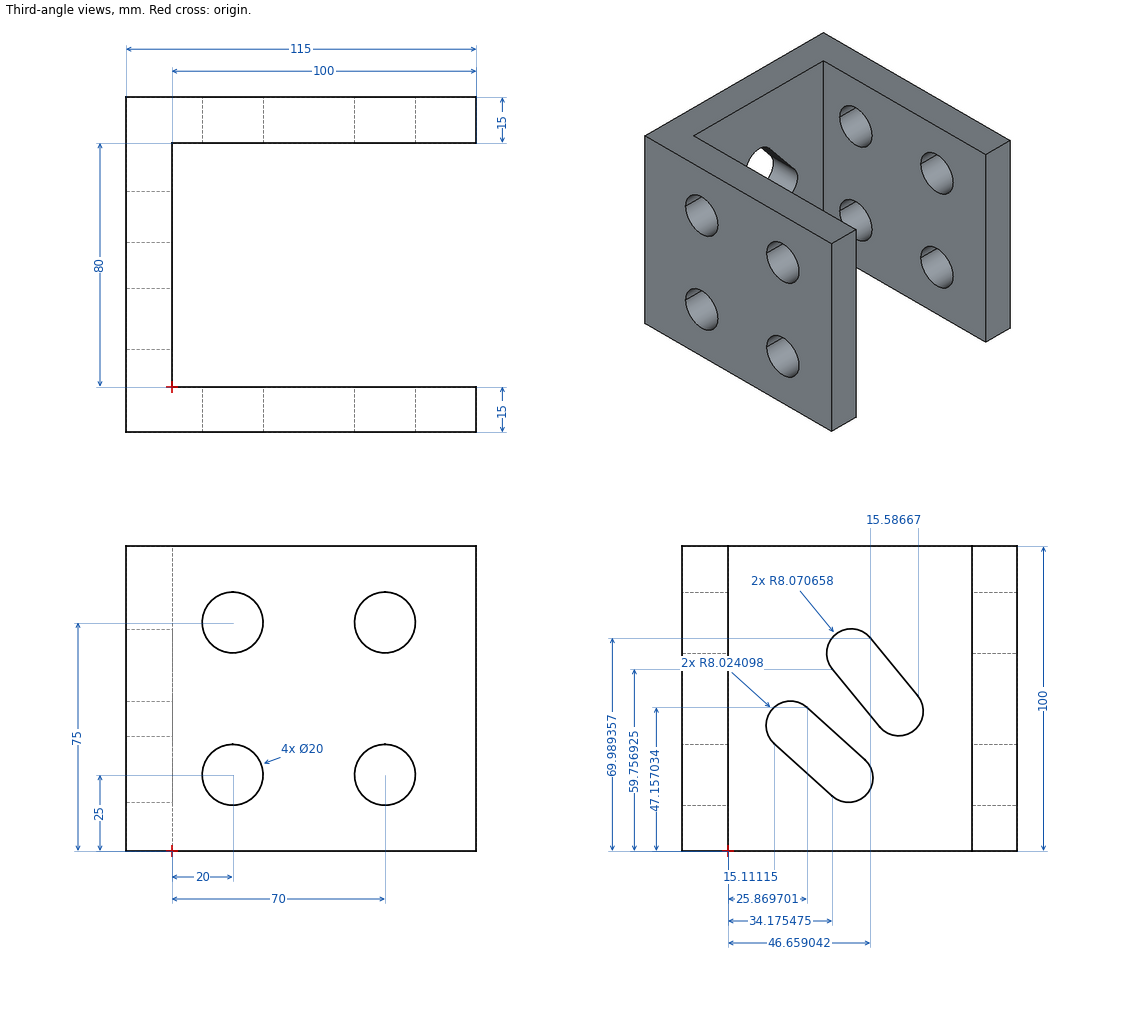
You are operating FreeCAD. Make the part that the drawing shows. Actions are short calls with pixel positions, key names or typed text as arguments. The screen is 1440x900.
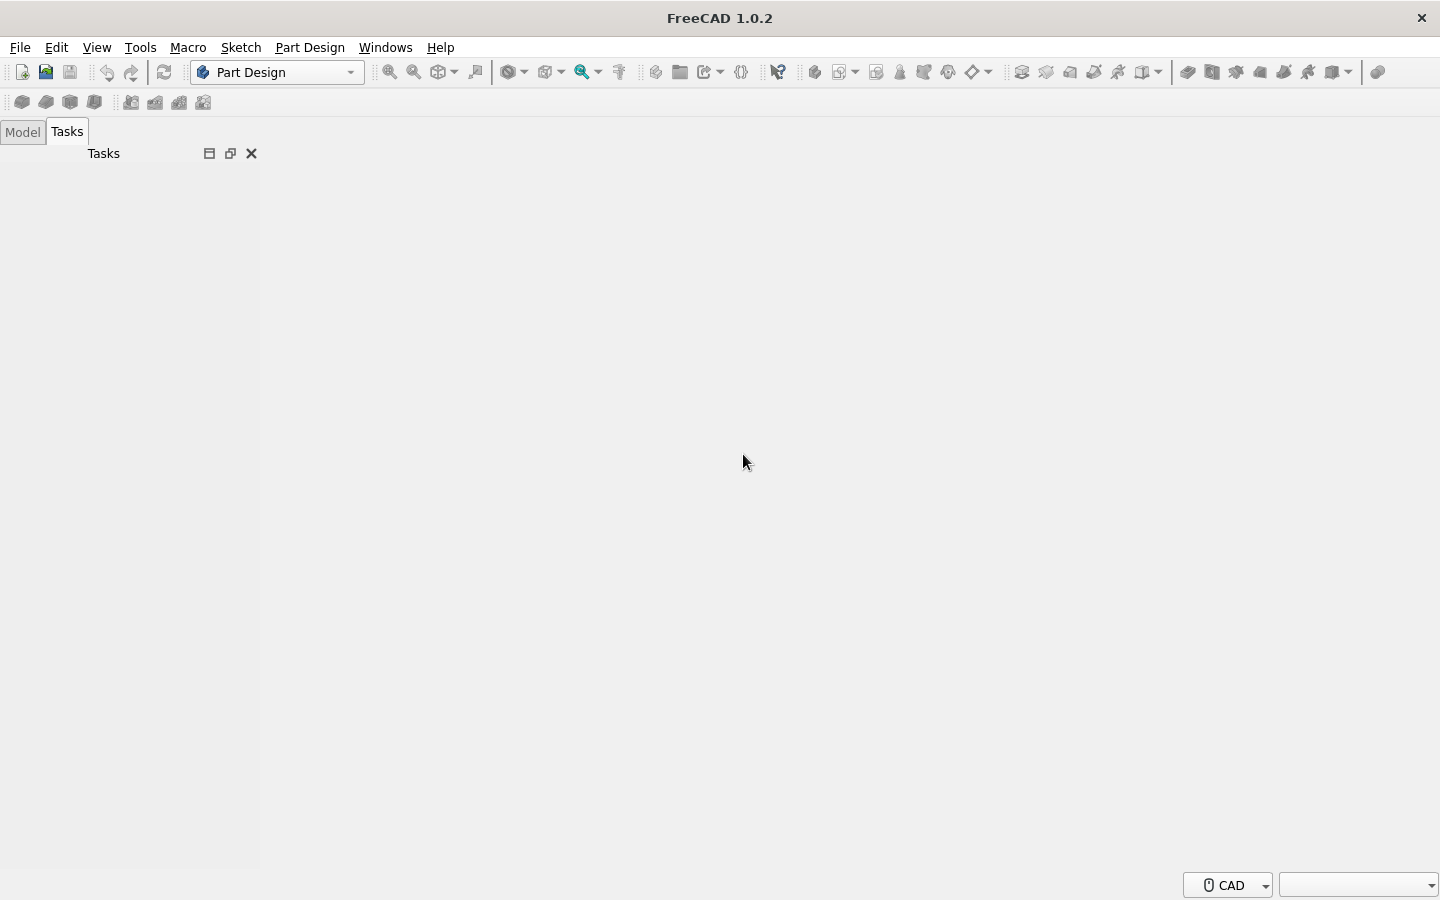
key(ctrl+n)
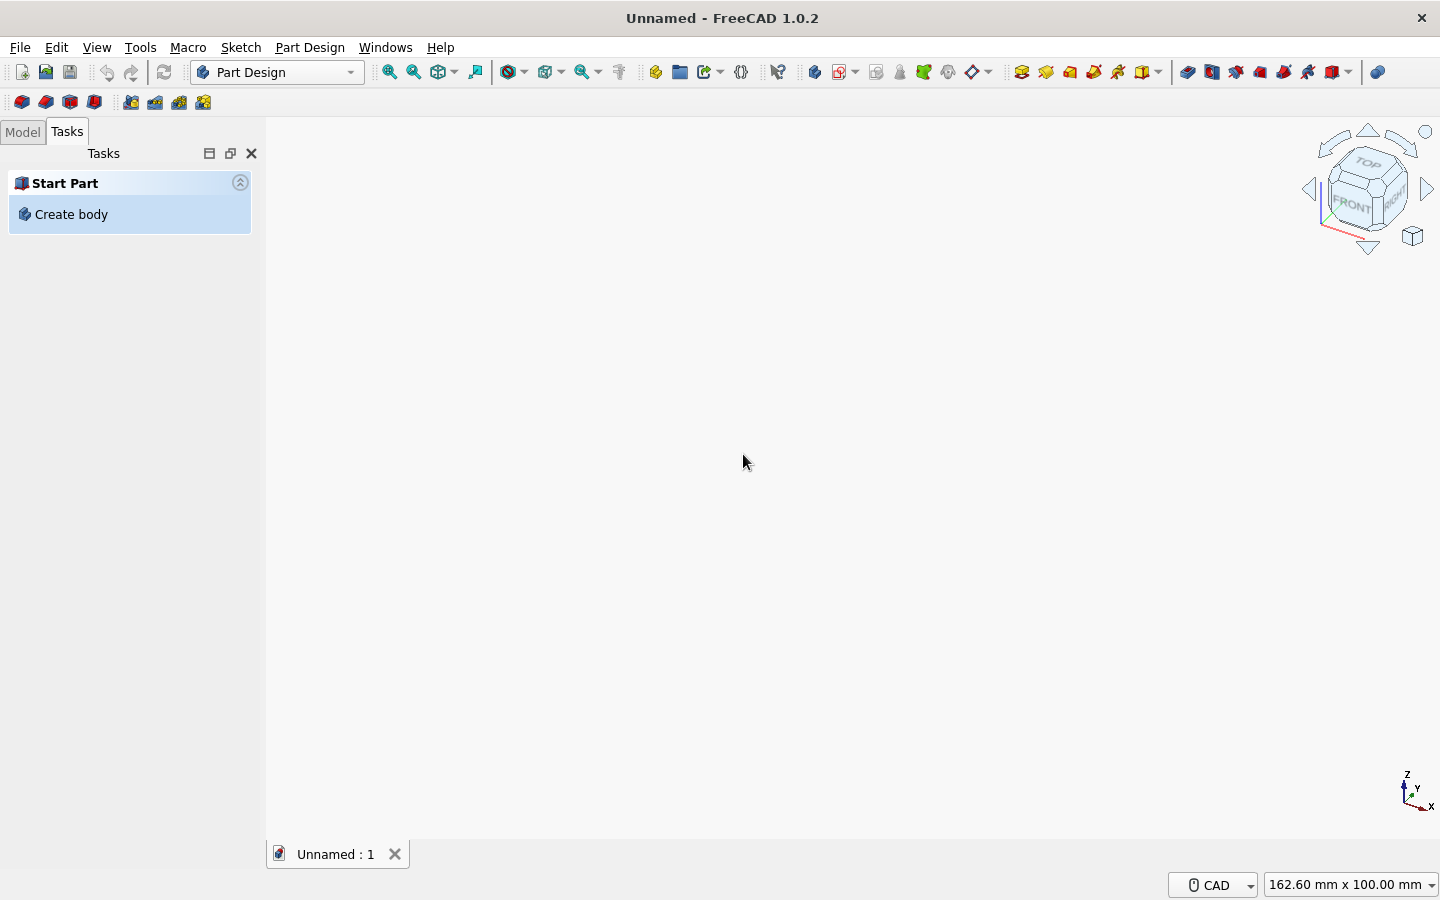
click(840, 72)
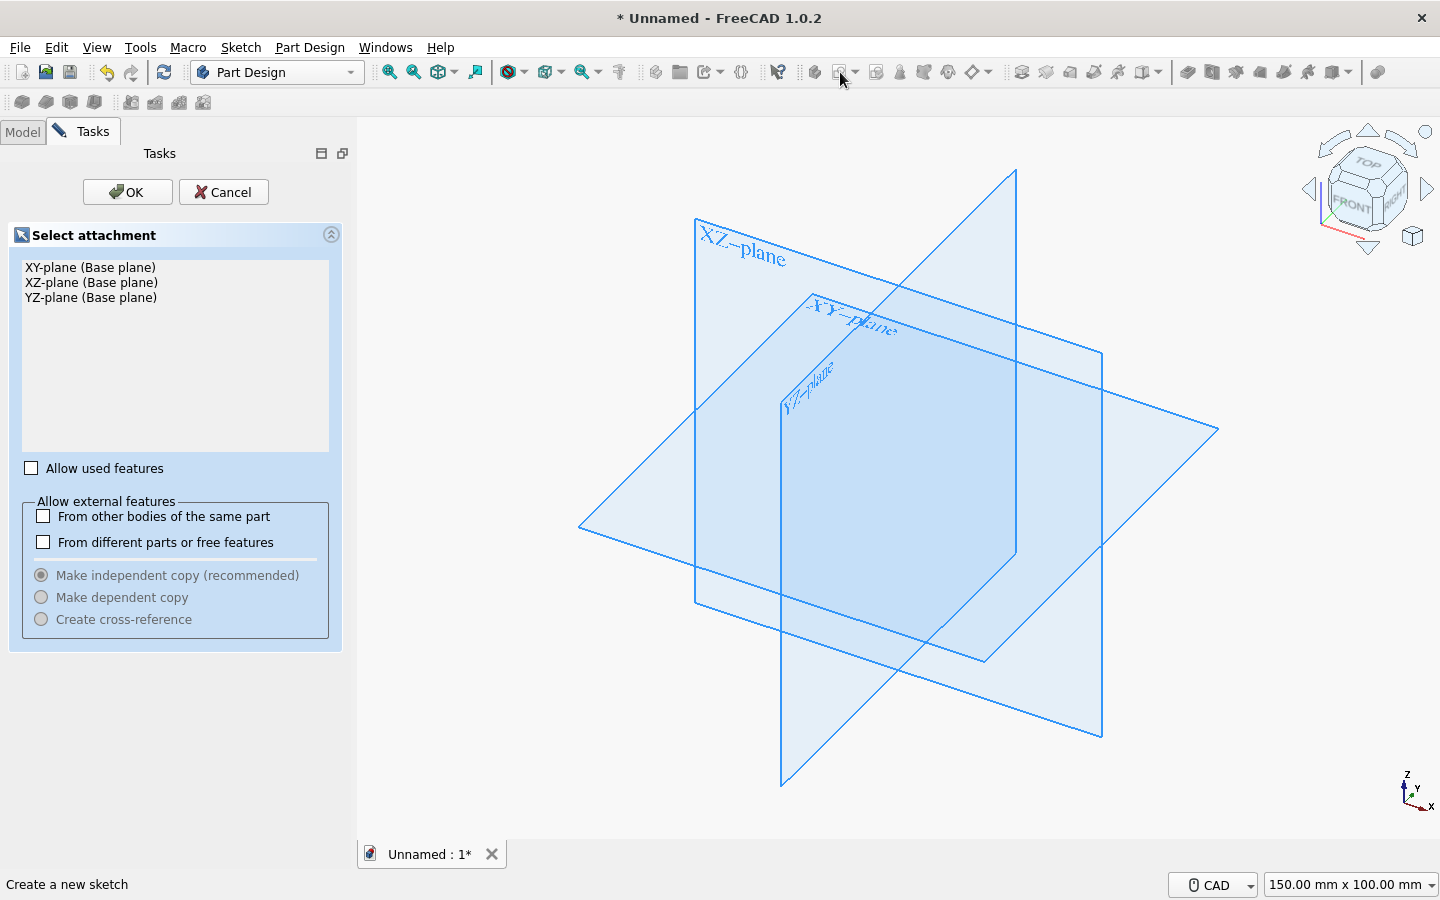
click(82, 268)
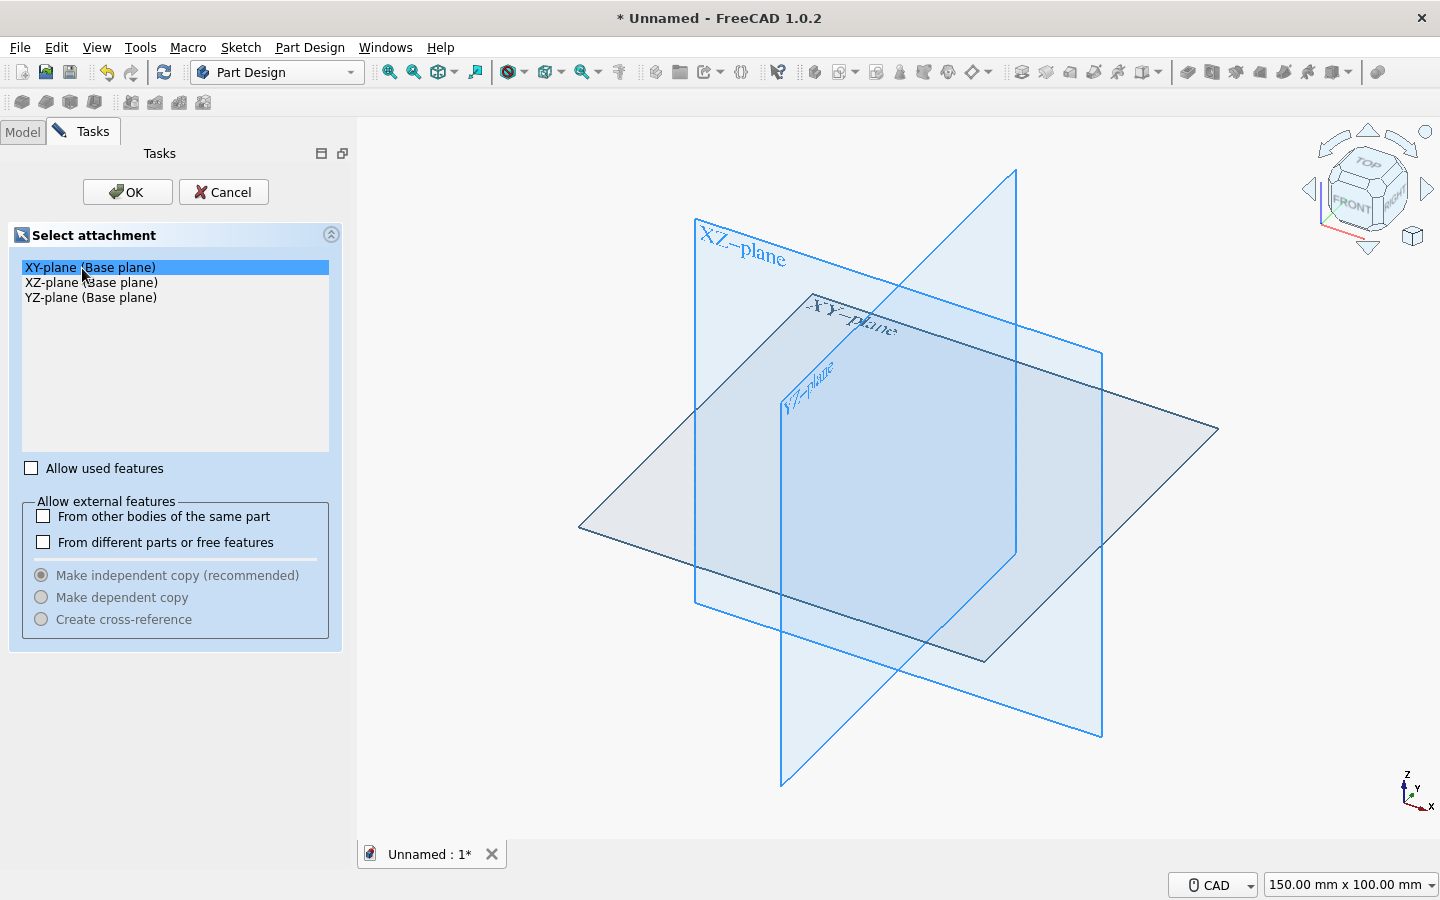
click(128, 192)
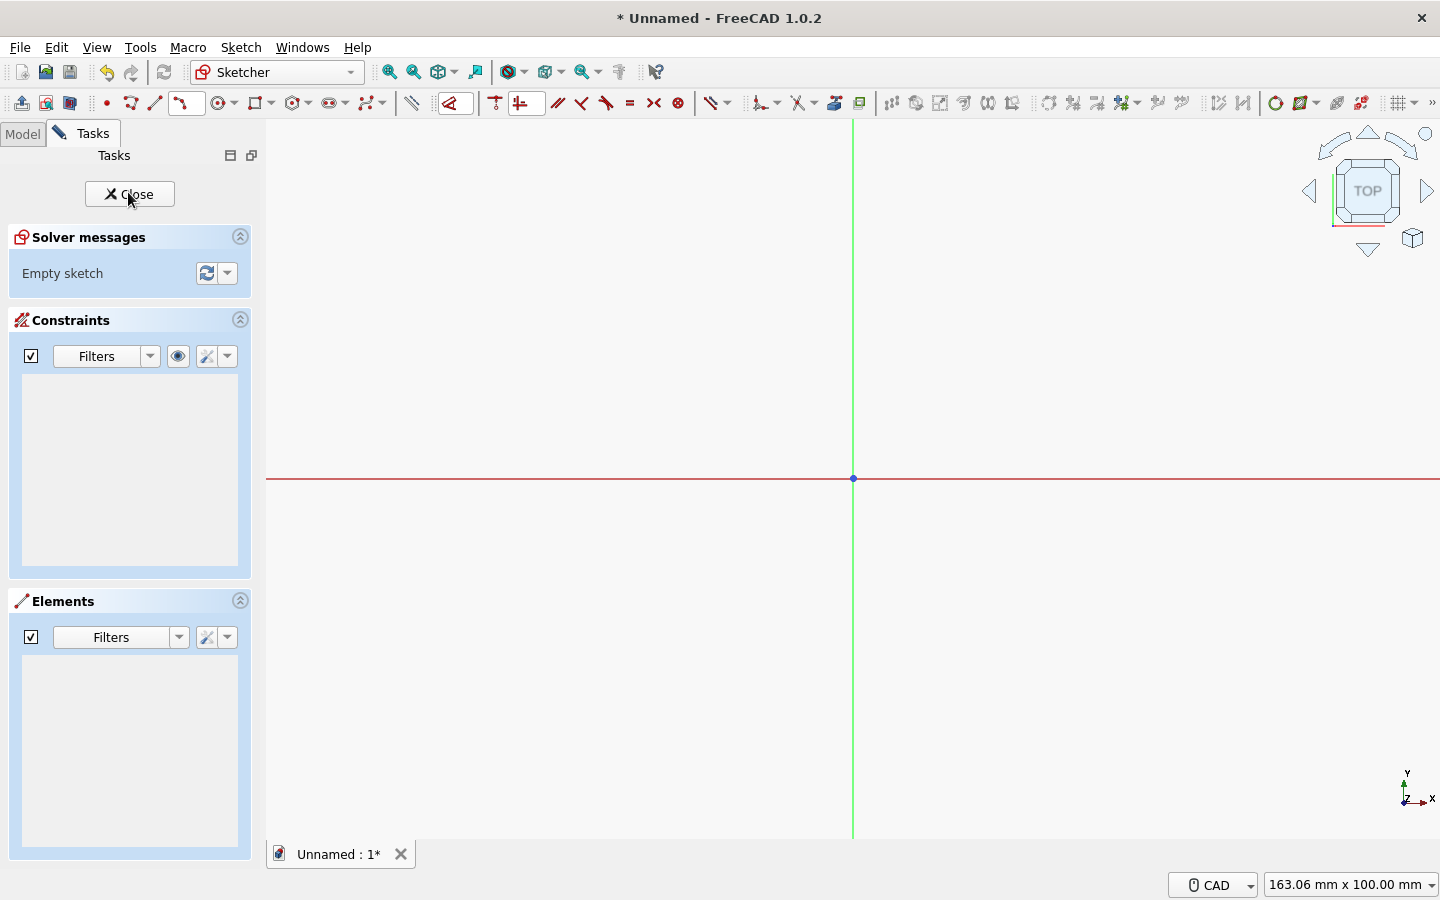
scroll(329, 811, down, 3)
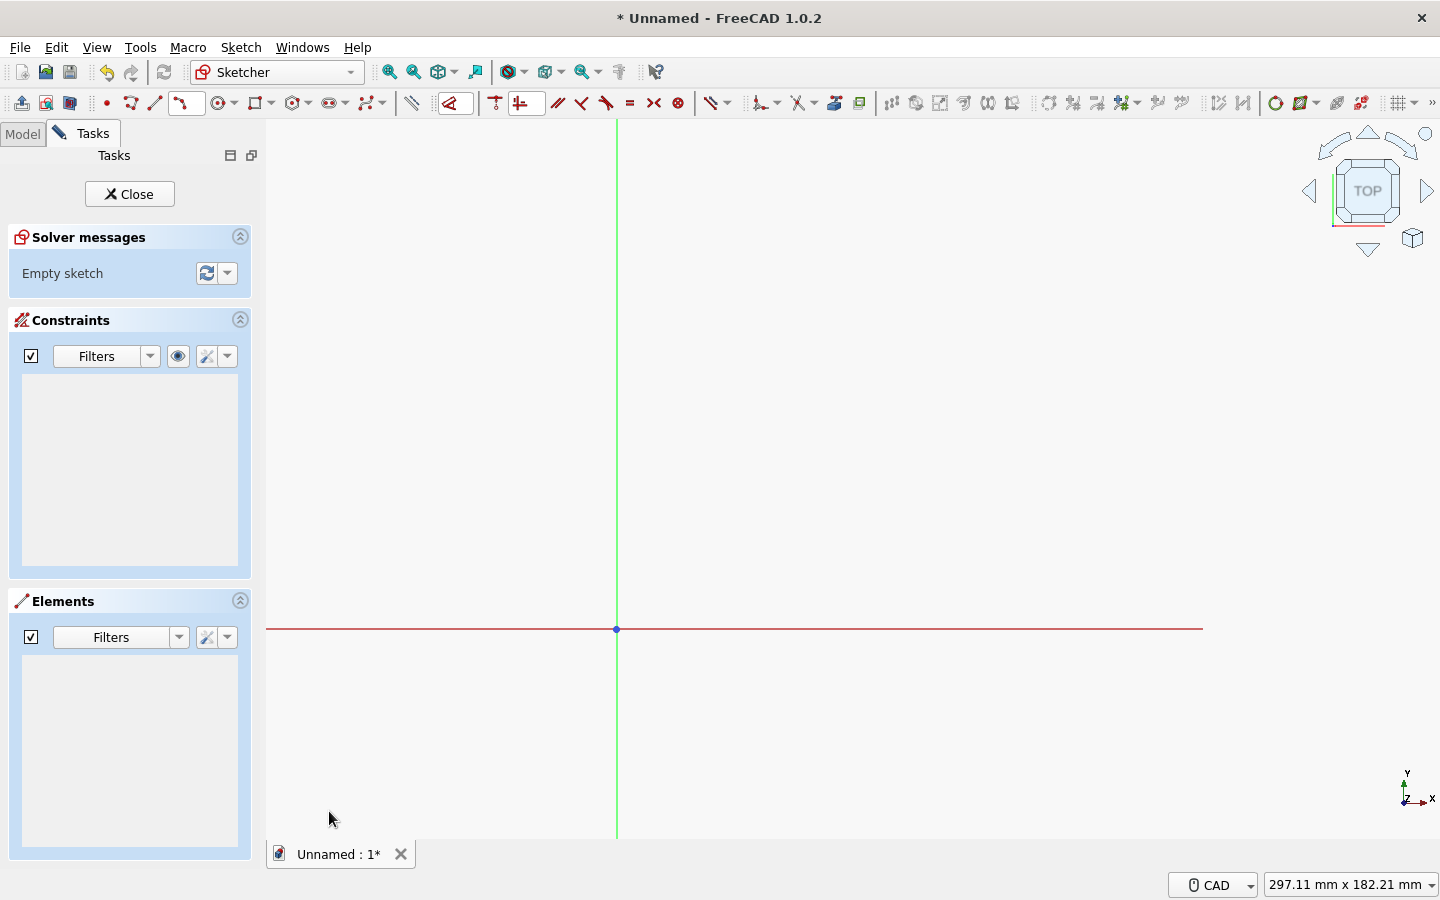
key(g)
key(m)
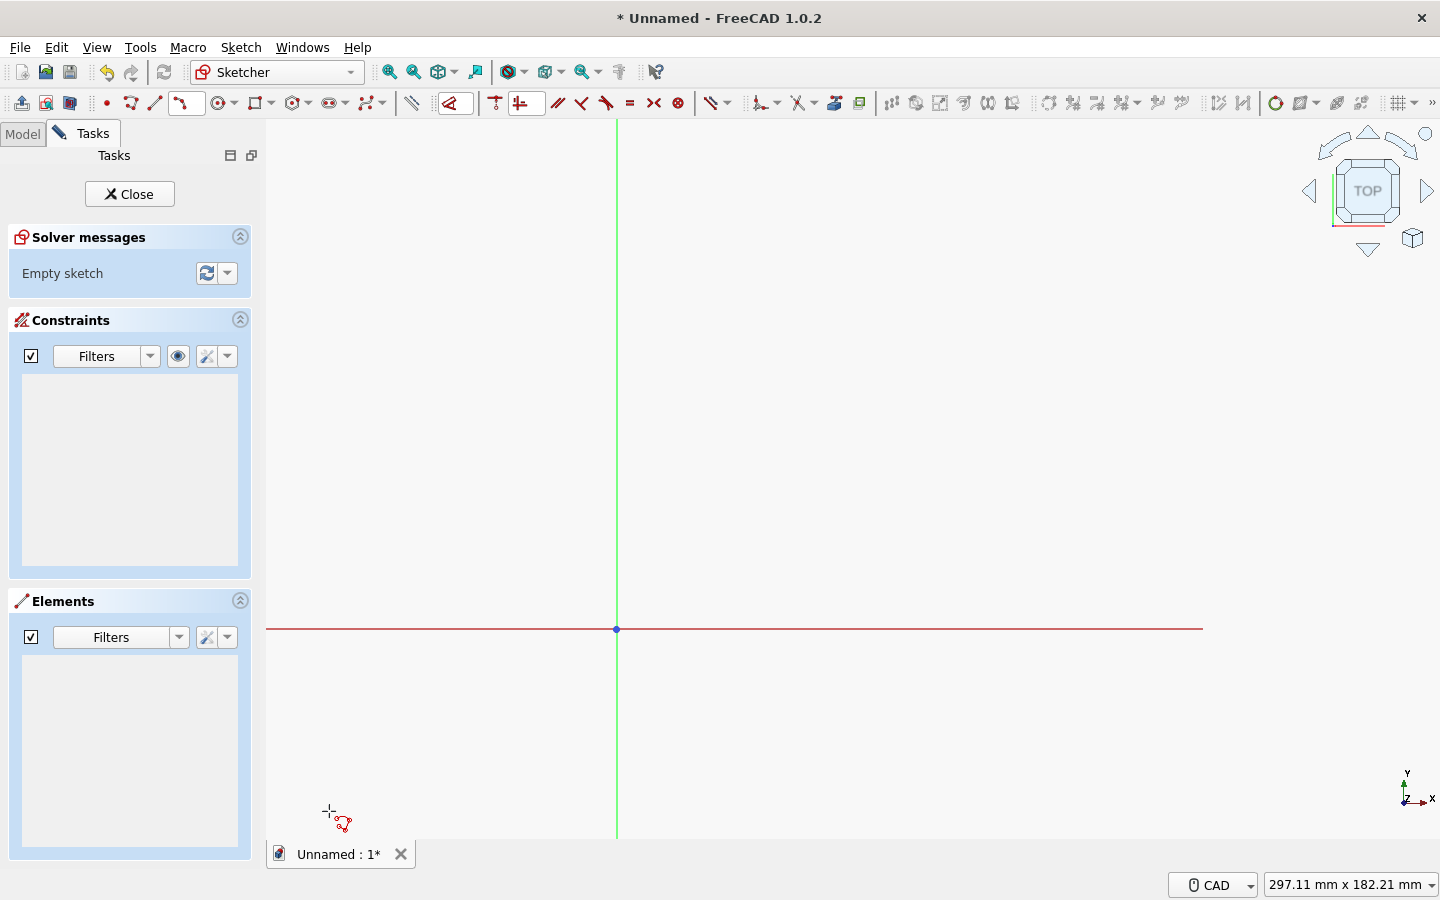
click(617, 629)
click(626, 313)
click(1012, 313)
click(1012, 254)
click(557, 254)
click(557, 689)
click(1012, 689)
click(1012, 620)
click(617, 629)
key(Escape)
key(Escape)